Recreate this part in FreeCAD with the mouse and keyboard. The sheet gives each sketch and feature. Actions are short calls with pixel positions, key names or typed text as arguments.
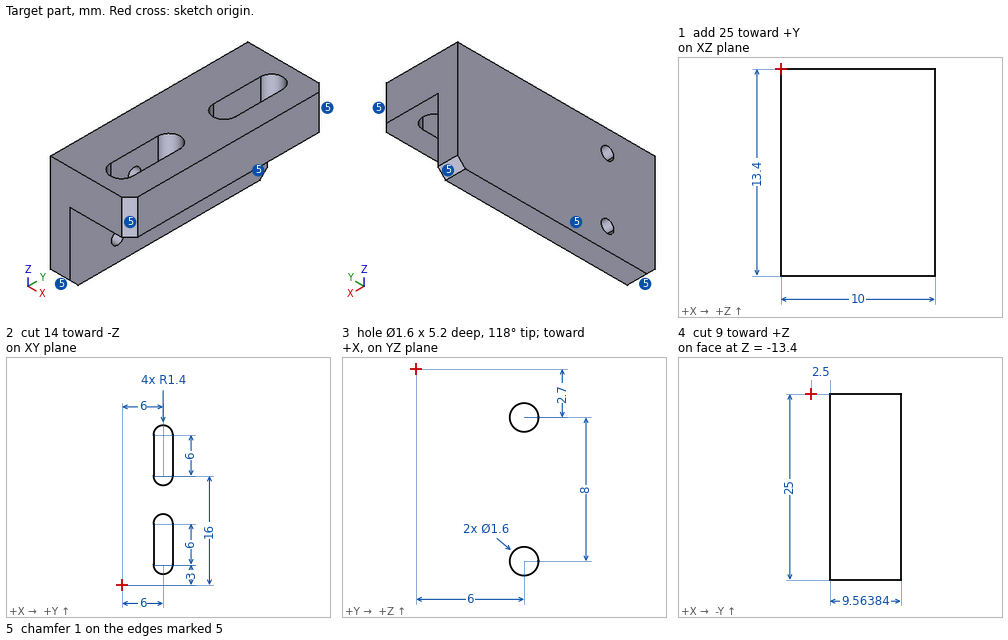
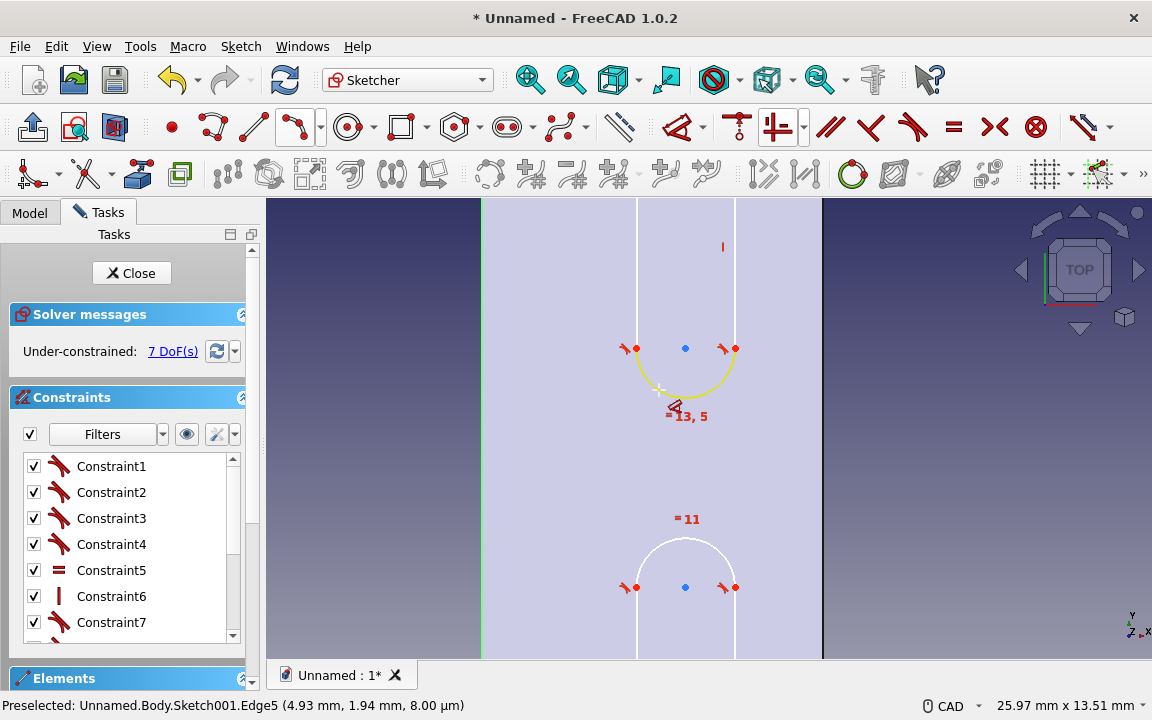
click(657, 389)
click(638, 415)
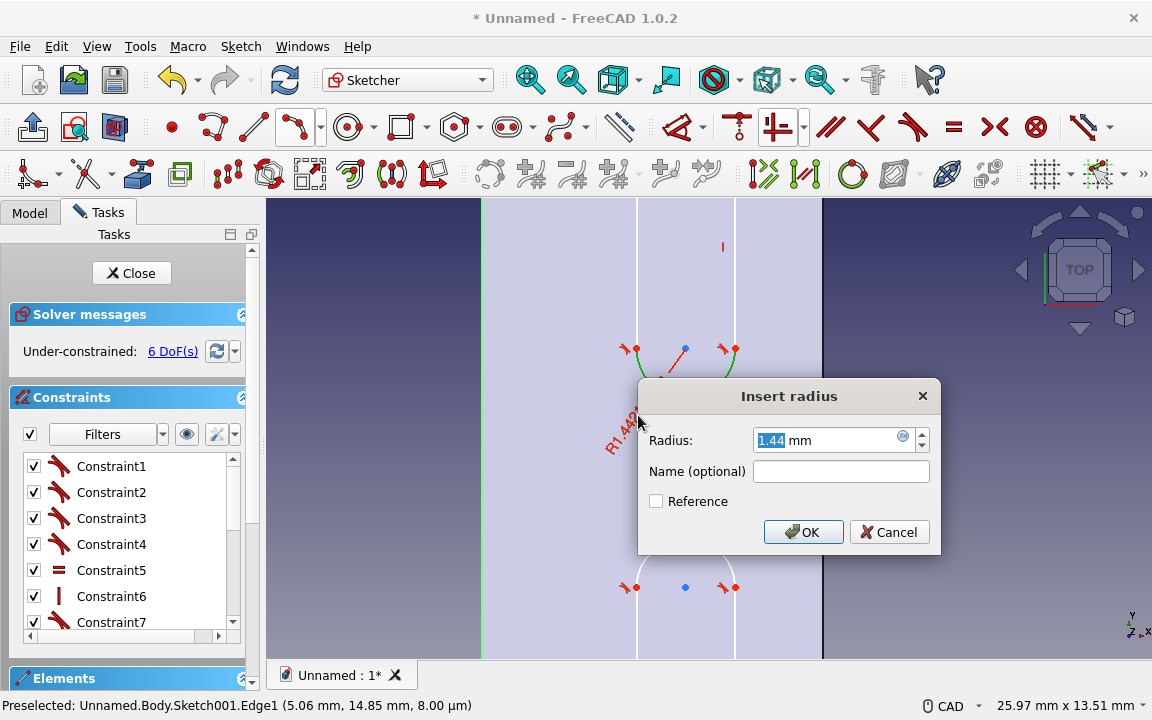
text(1.4)
key(Return)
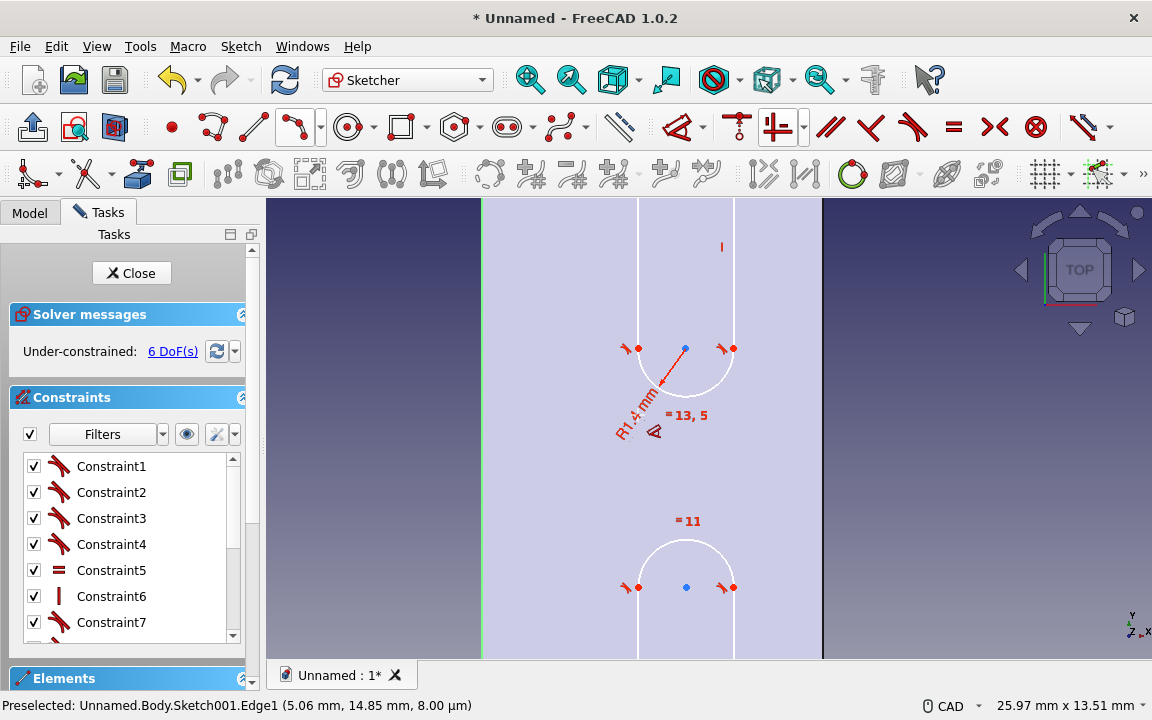
click(638, 288)
click(672, 287)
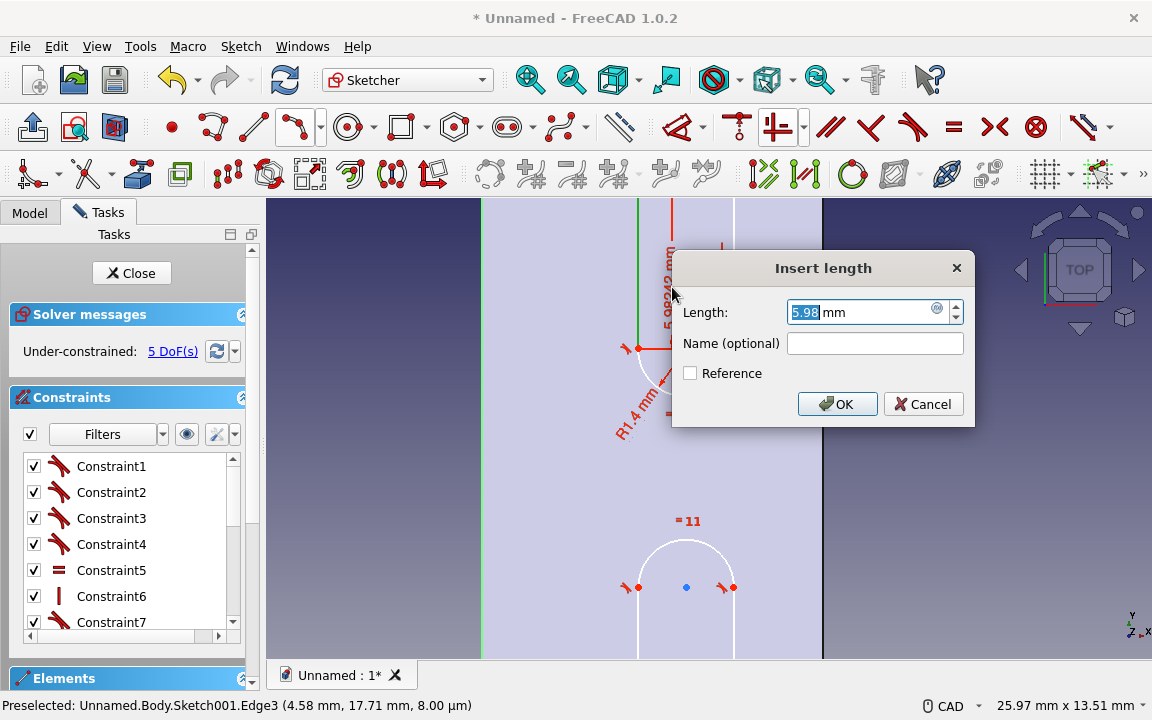
text(6)
key(Return)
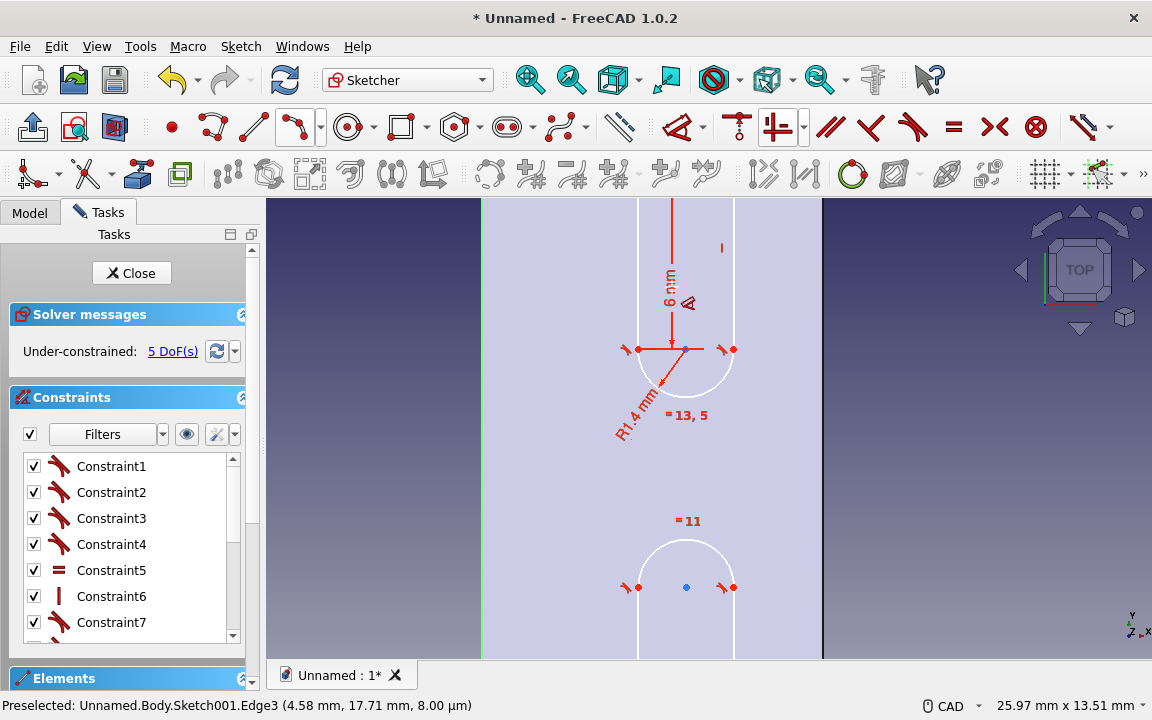
click(638, 629)
click(672, 609)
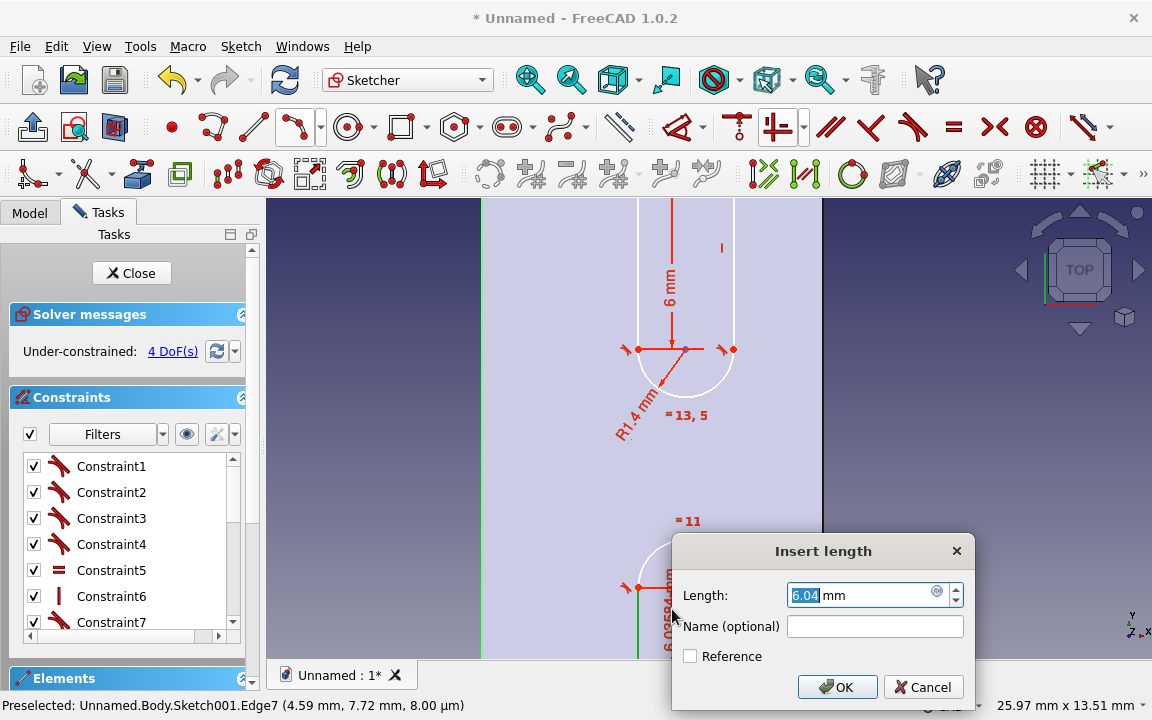
text(6)
key(Return)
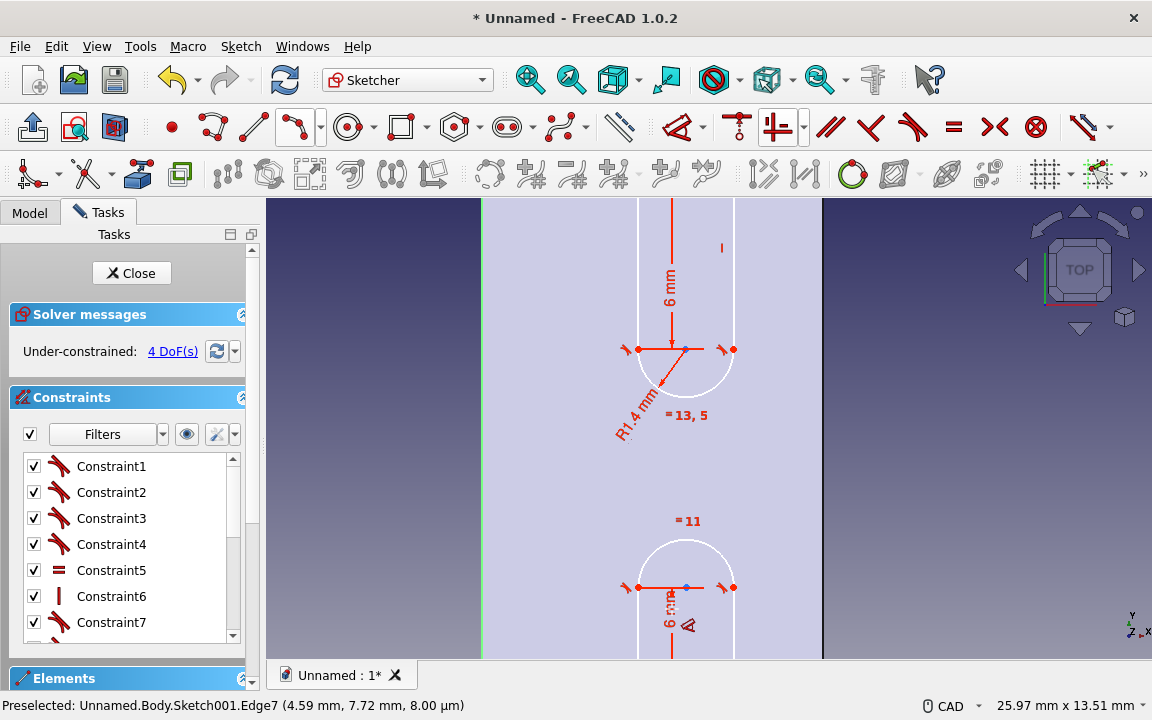
scroll(659, 390, down, 5)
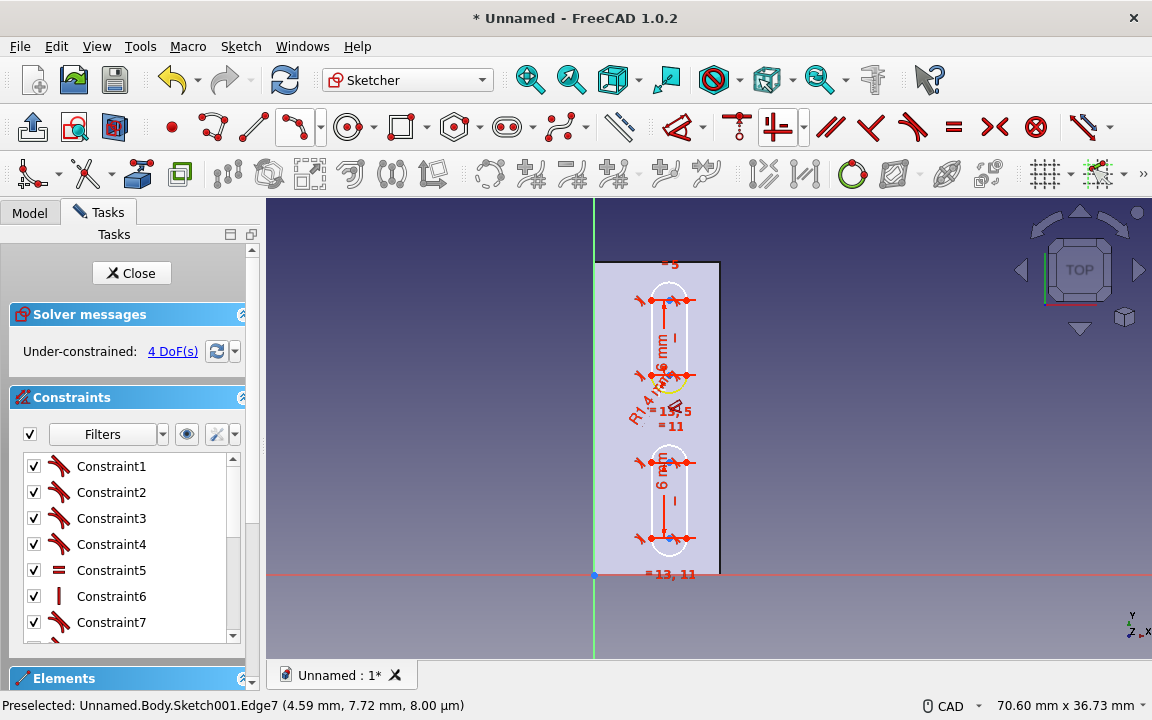
click(652, 538)
click(560, 557)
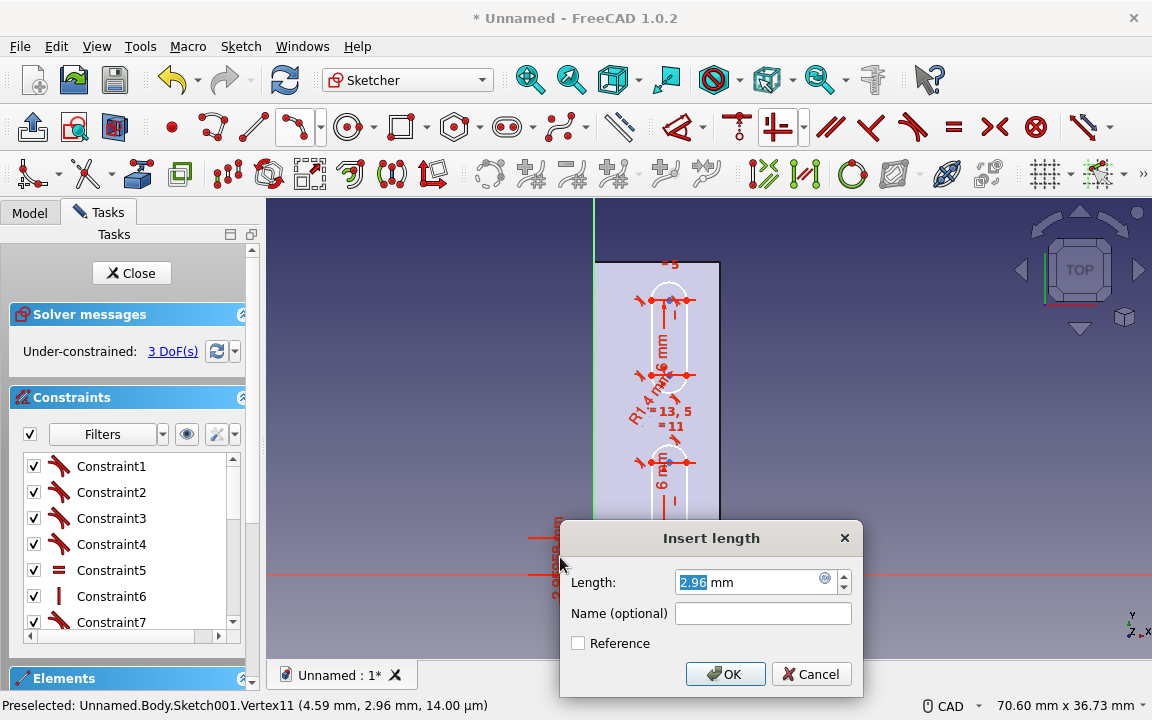
text(3)
key(Return)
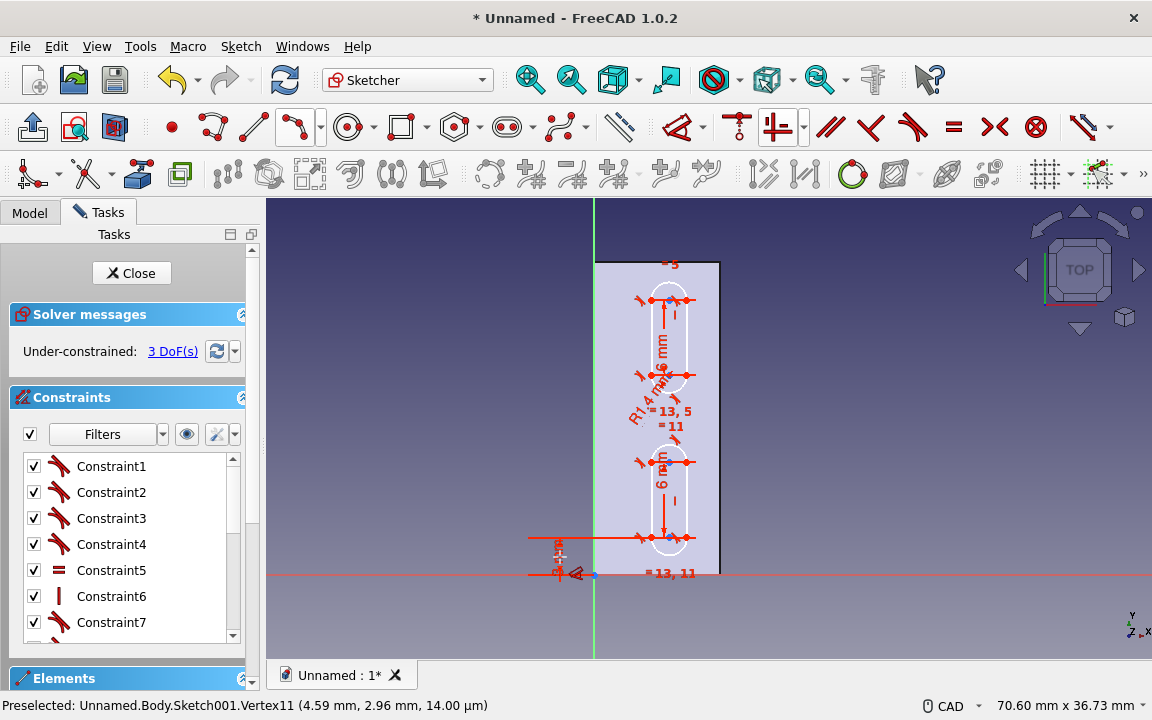
click(669, 375)
click(632, 609)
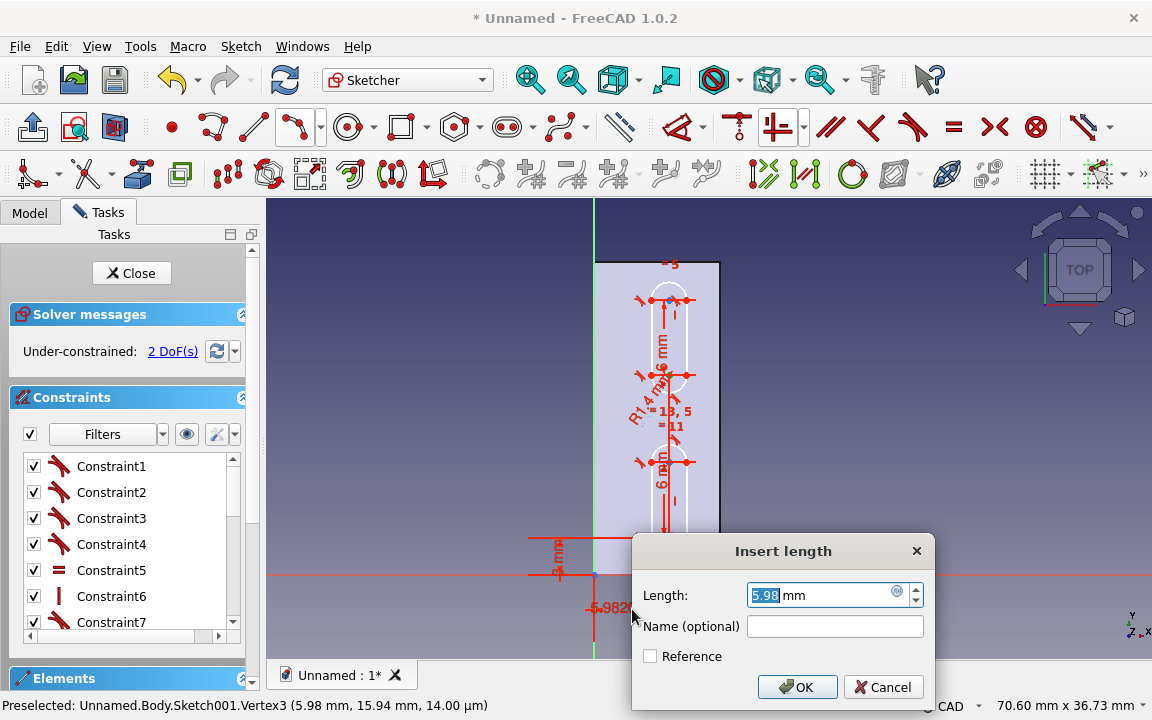
text(6)
key(Return)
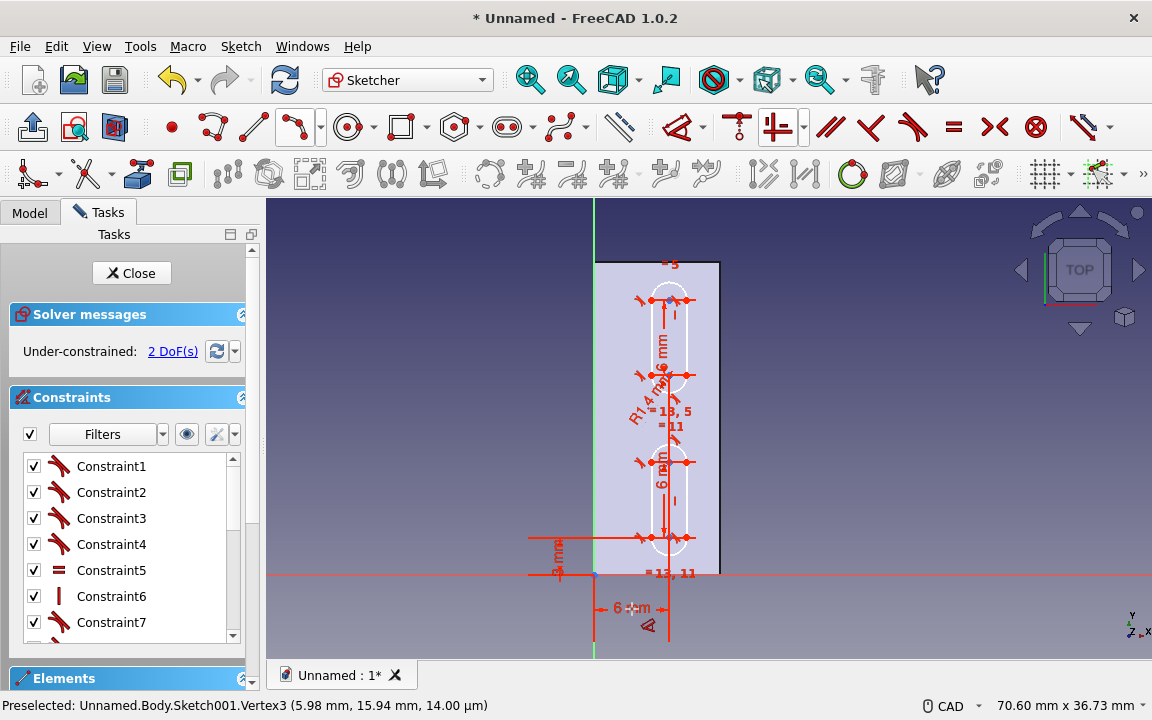
click(669, 538)
click(632, 504)